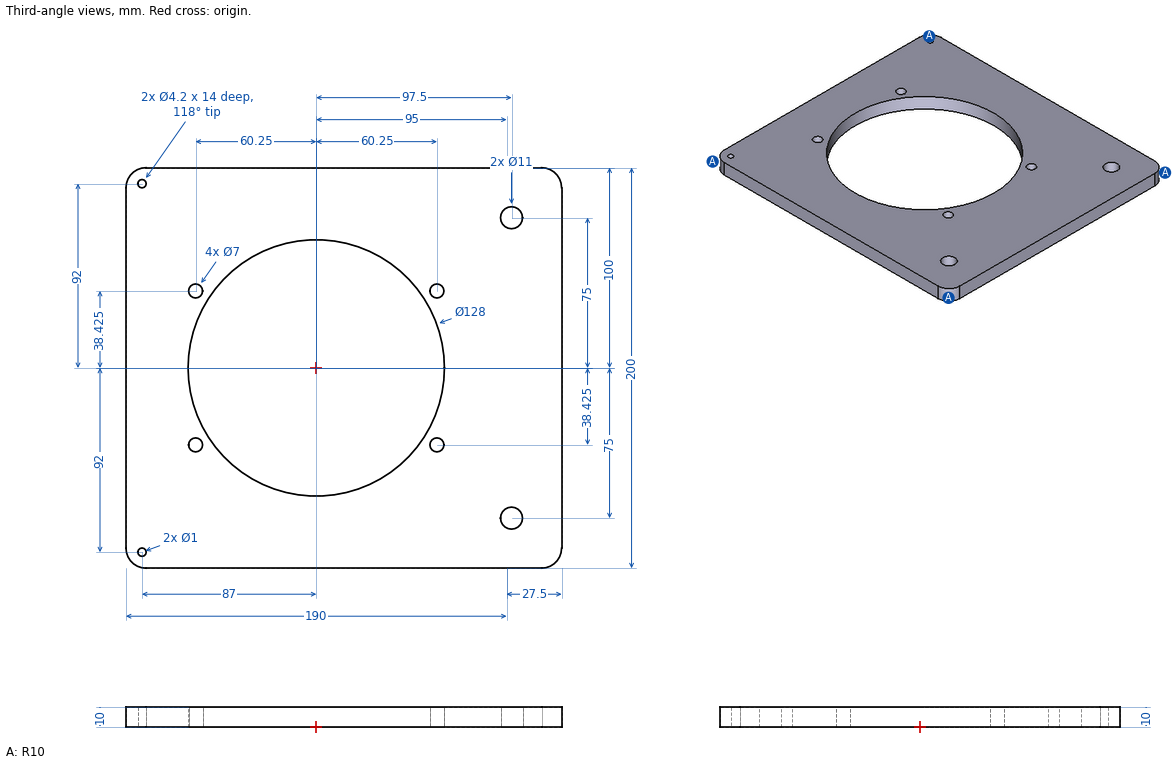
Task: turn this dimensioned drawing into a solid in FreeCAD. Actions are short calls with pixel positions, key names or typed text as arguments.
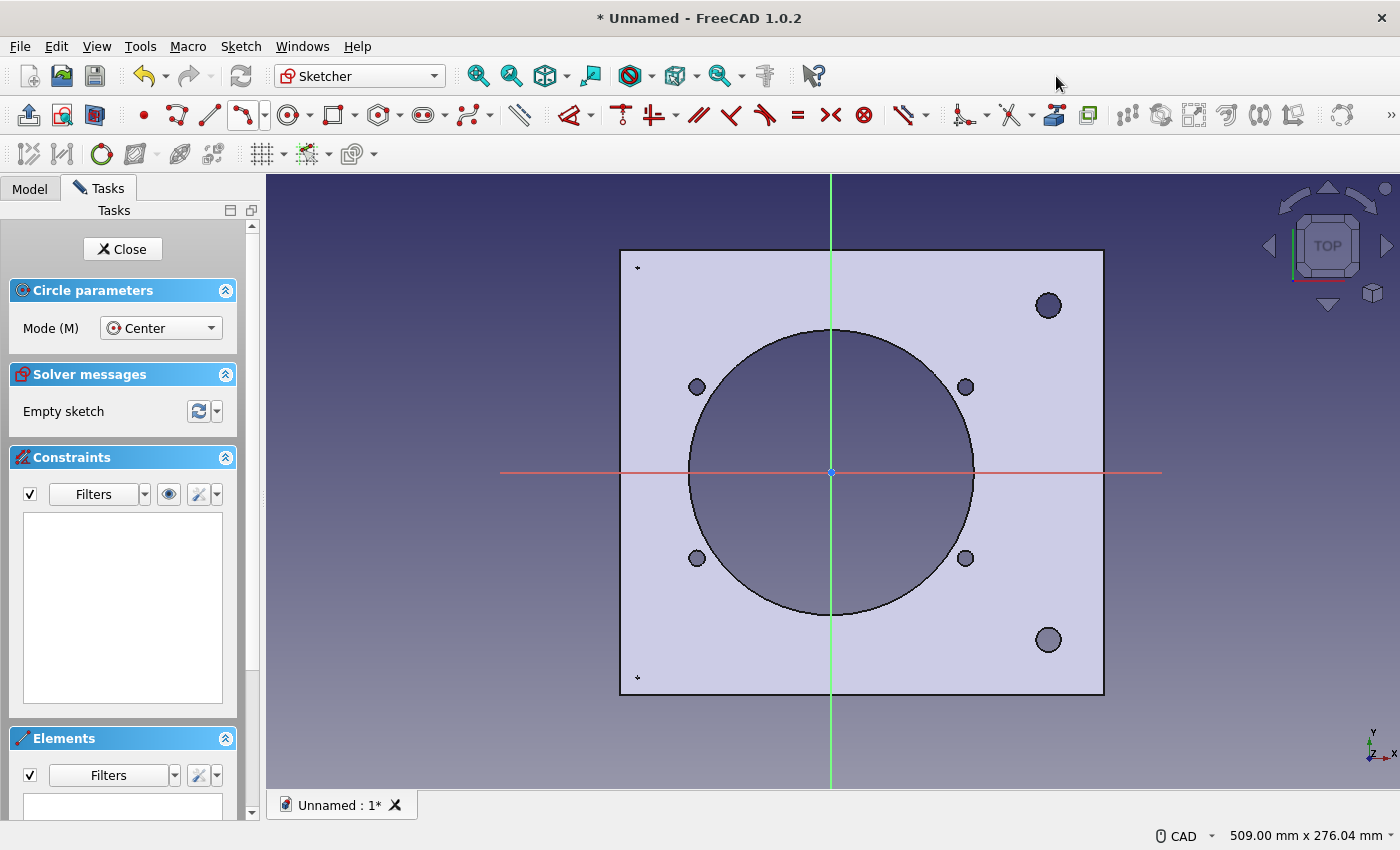
scroll(637, 268, up, 8)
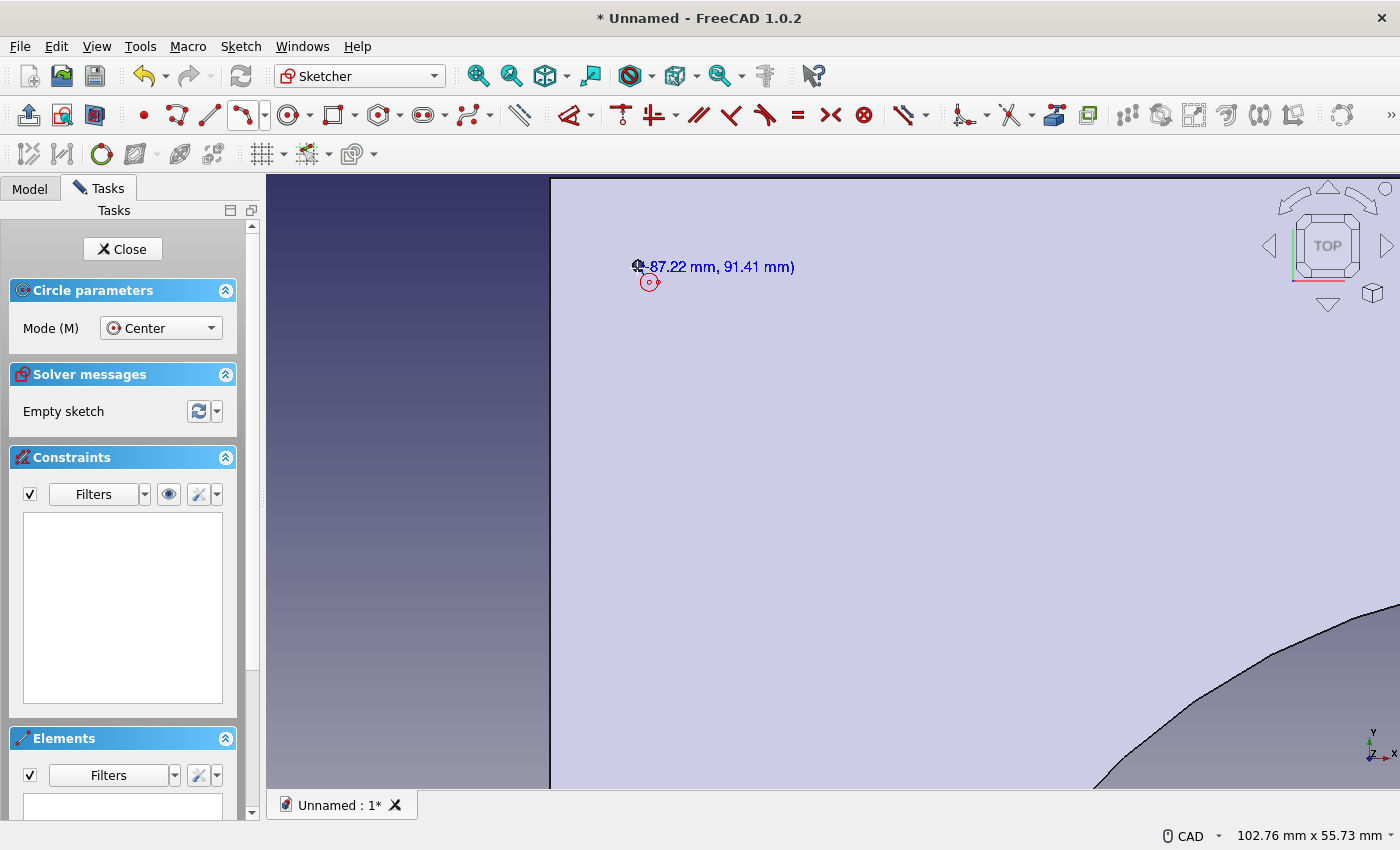
scroll(678, 279, down, 8)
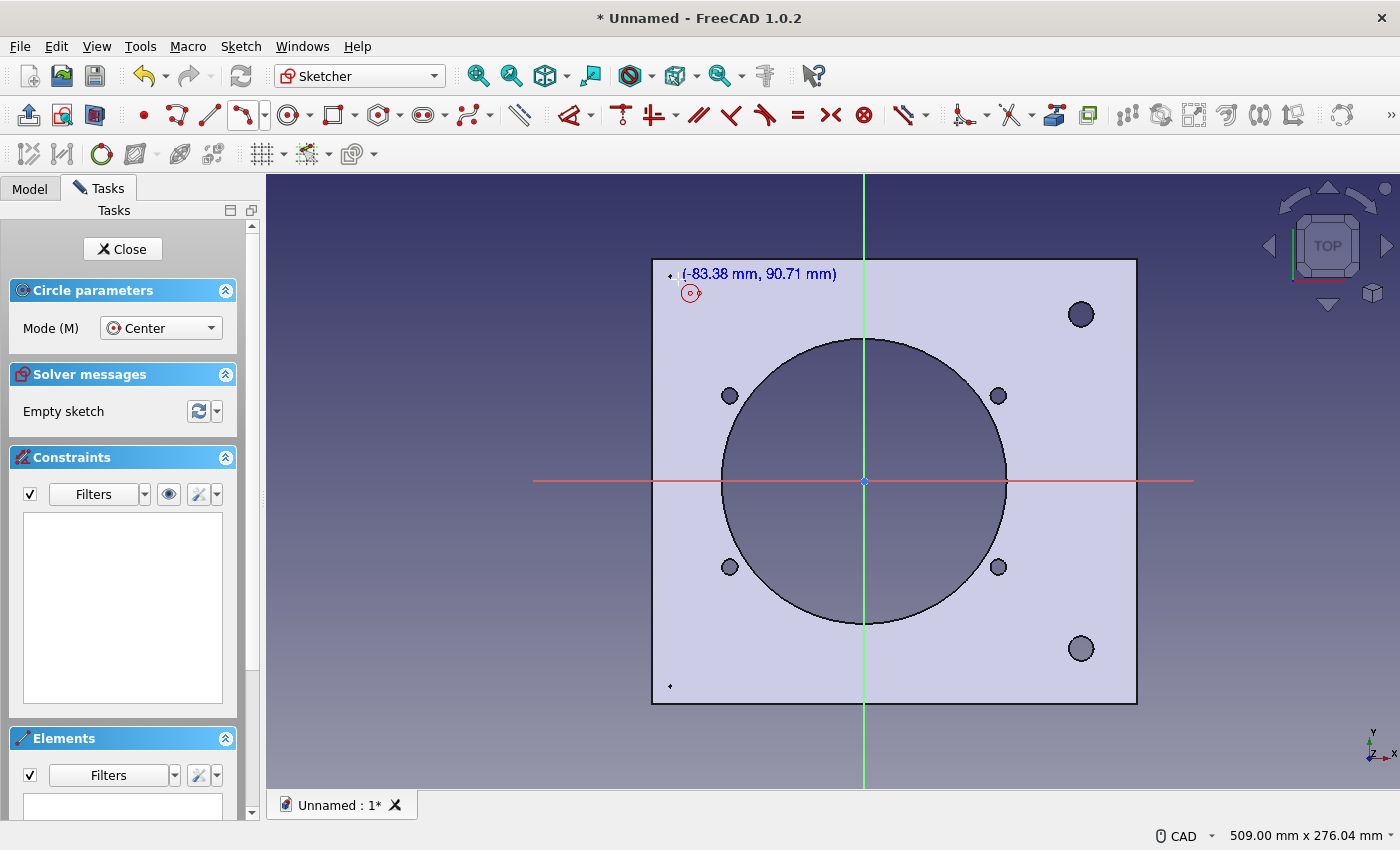
click(670, 276)
move(674, 273)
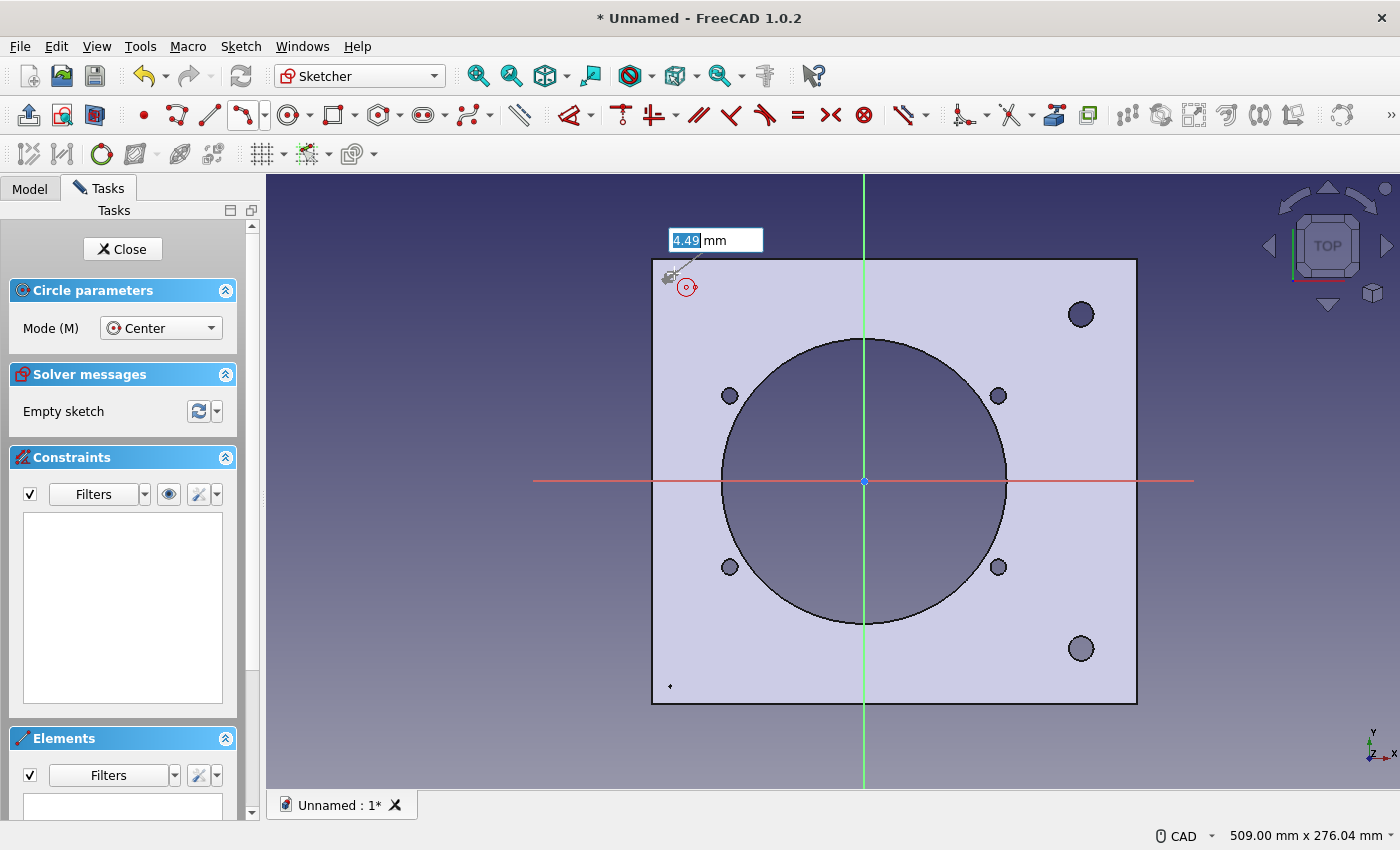
text(4.2)
key(Return)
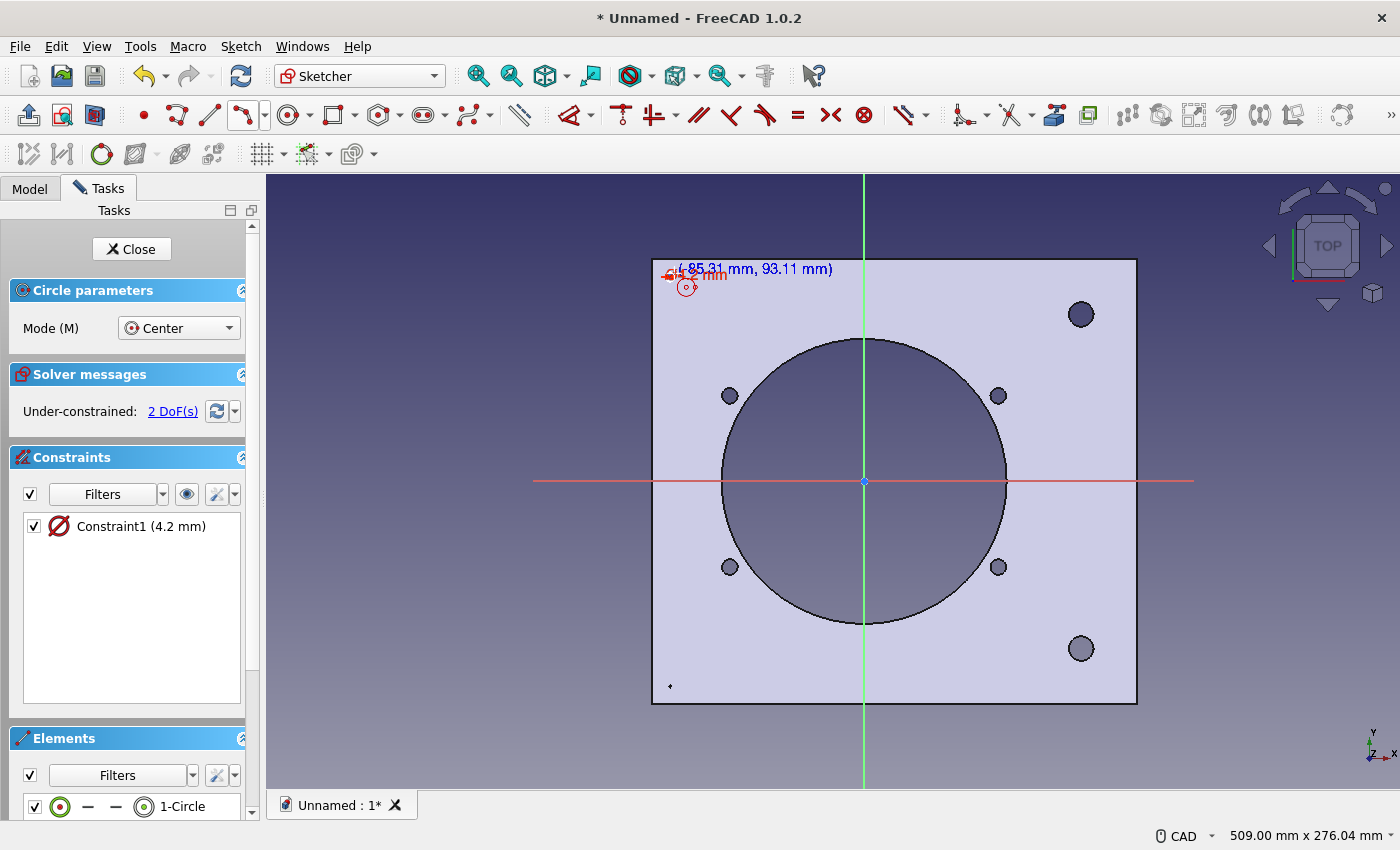
scroll(670, 686, up, 8)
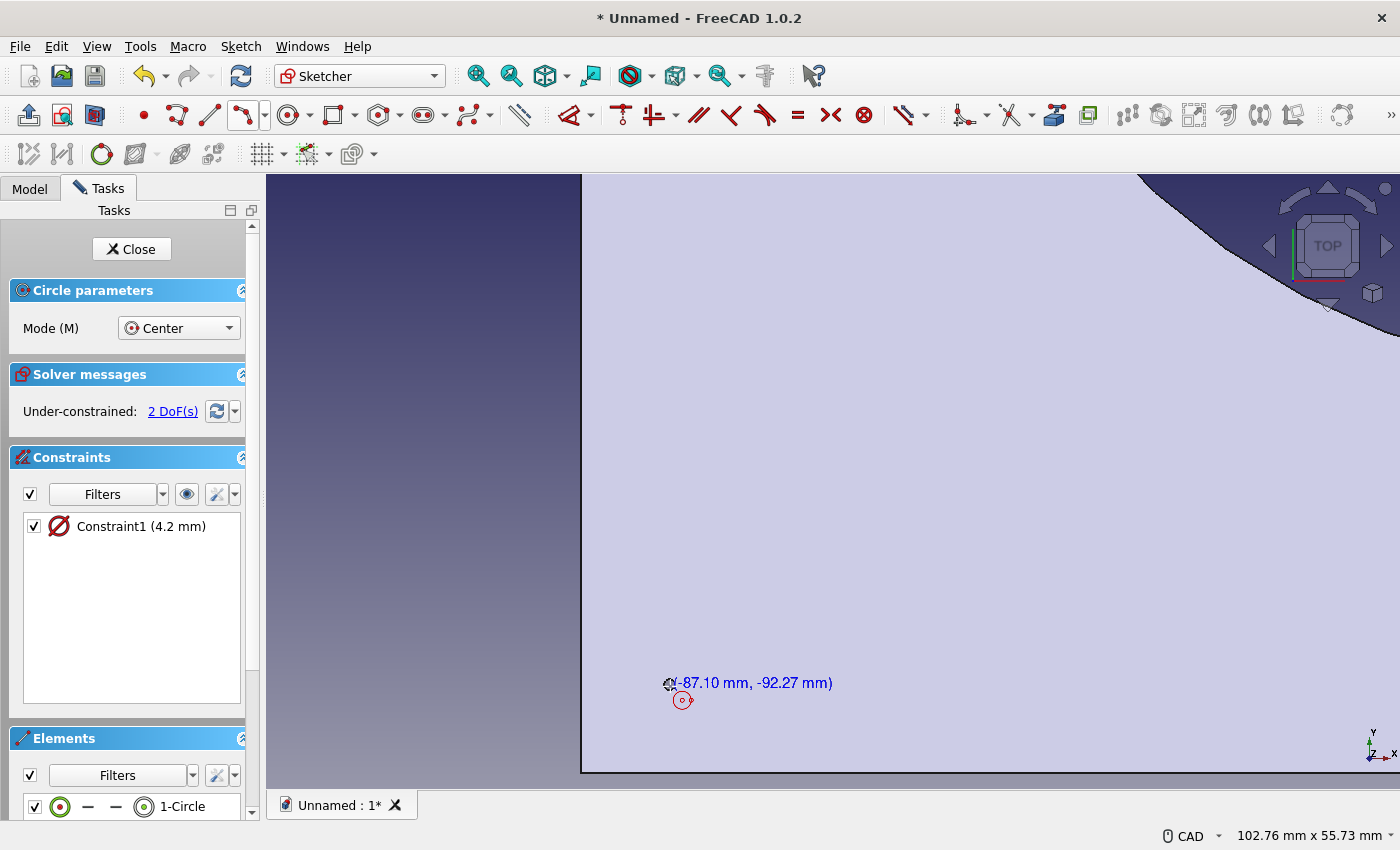
scroll(670, 687, down, 8)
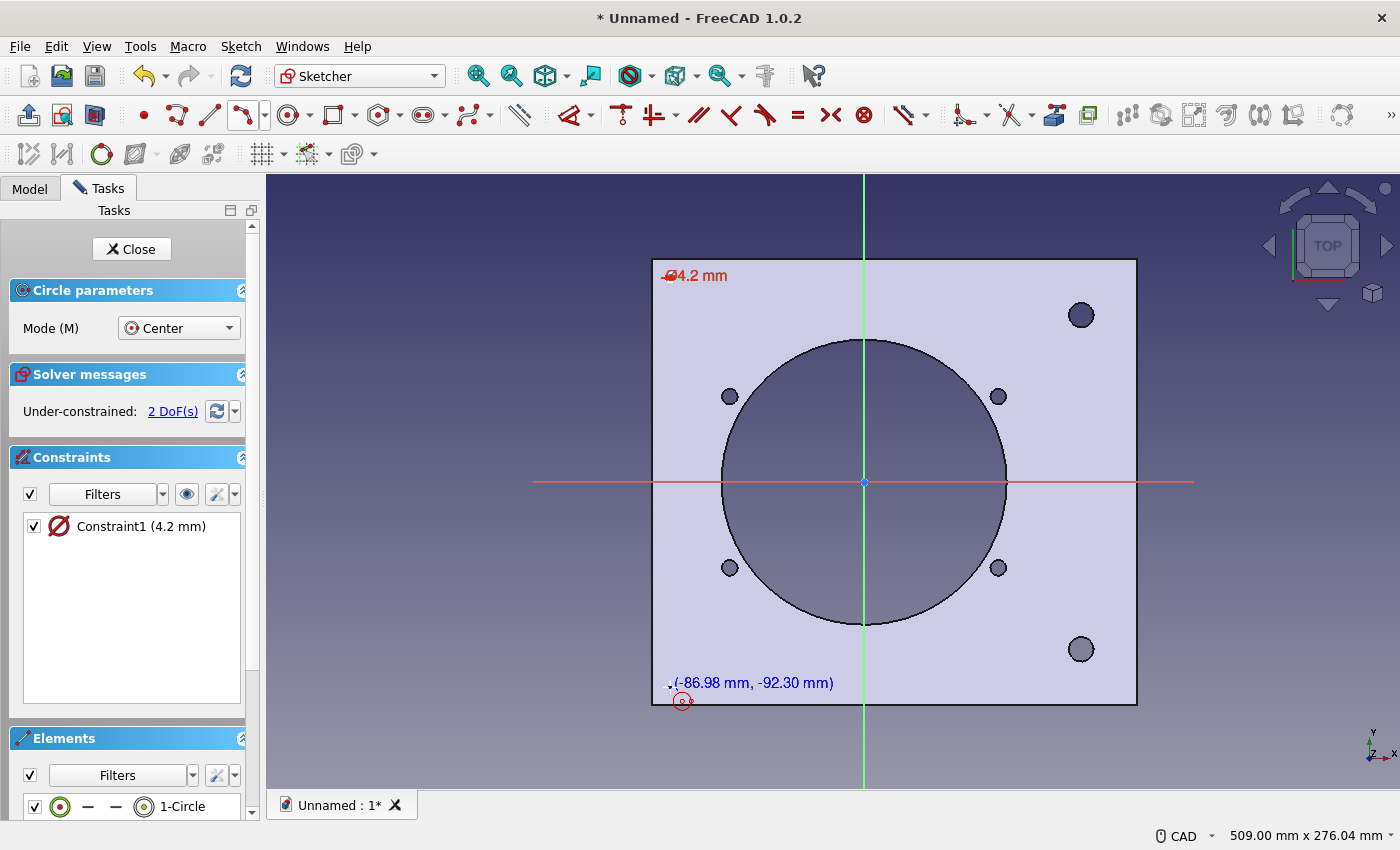
click(670, 687)
move(674, 684)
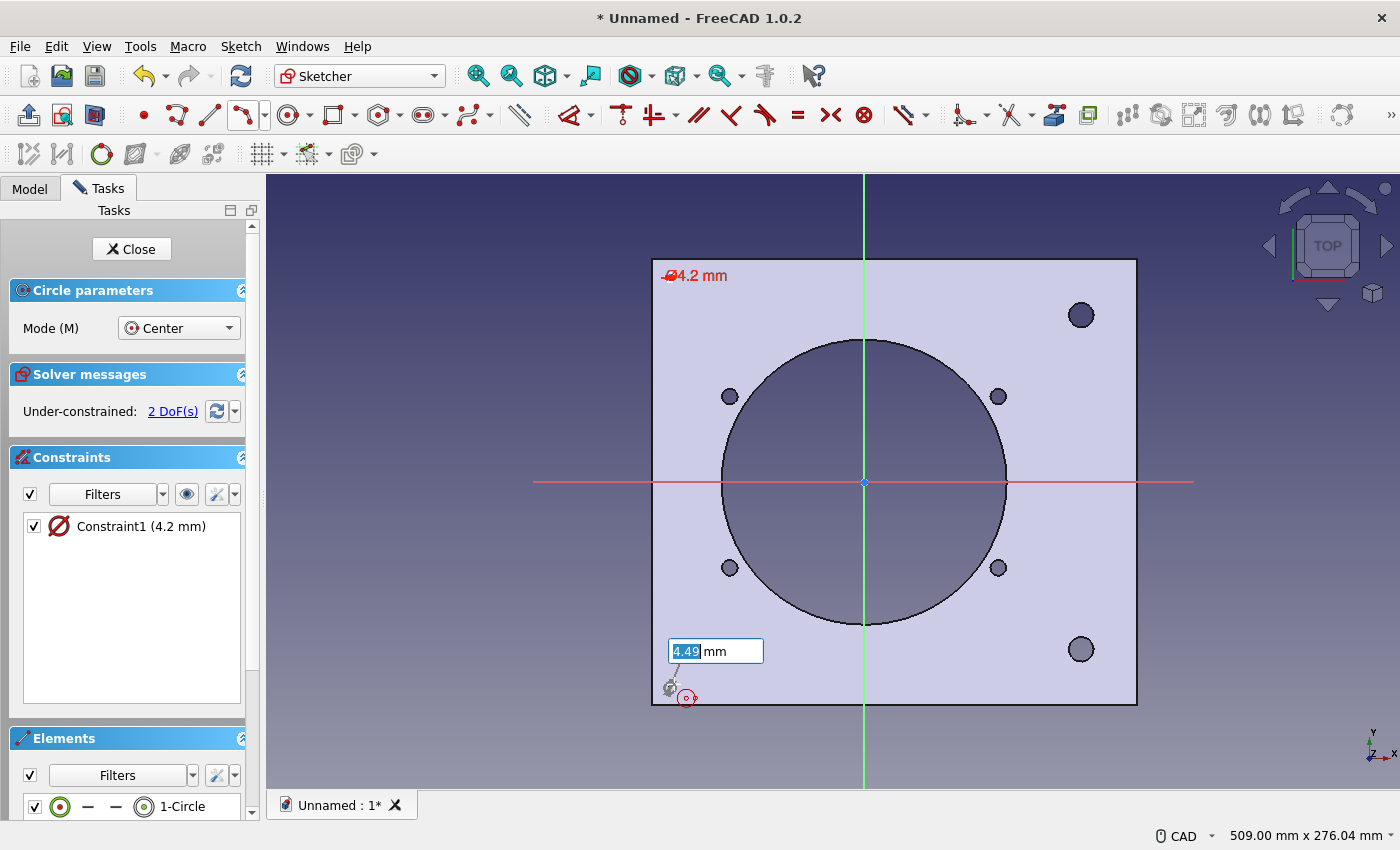
text(4.2)
key(Return)
key(Escape)